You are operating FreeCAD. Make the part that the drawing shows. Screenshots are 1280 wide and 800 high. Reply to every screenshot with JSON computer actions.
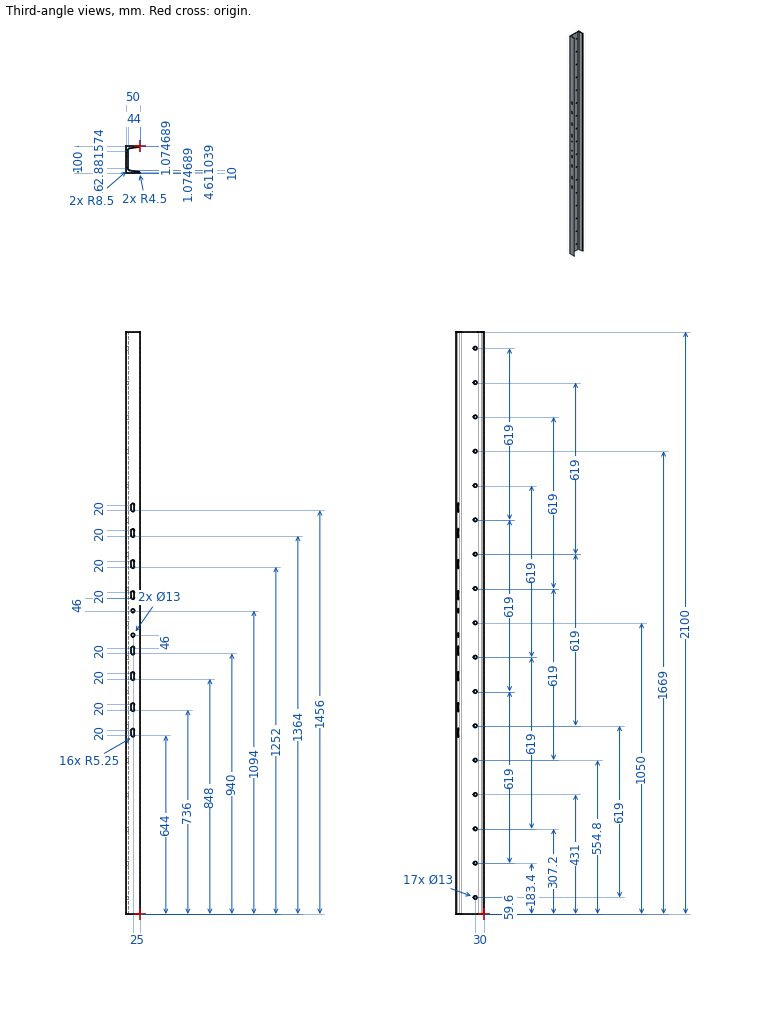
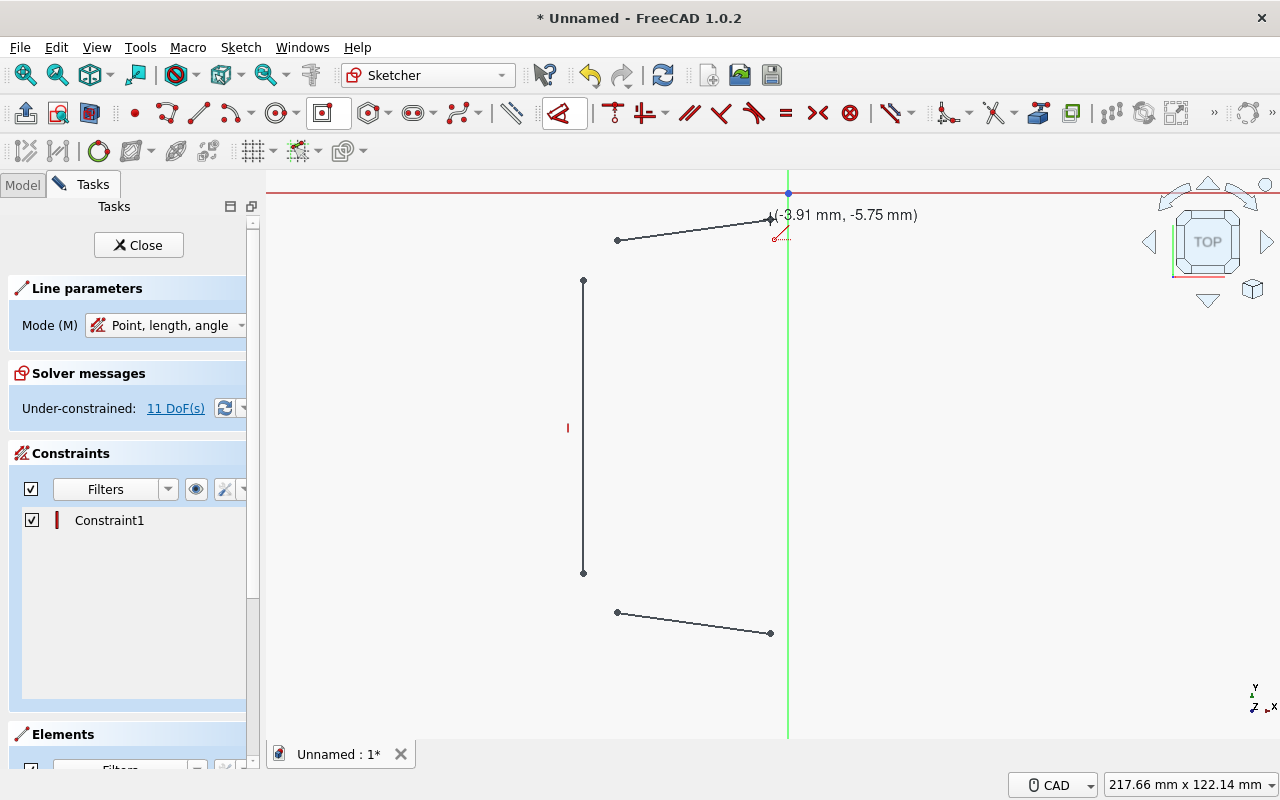
{"action": "left_click", "coordinate": [168, 114]}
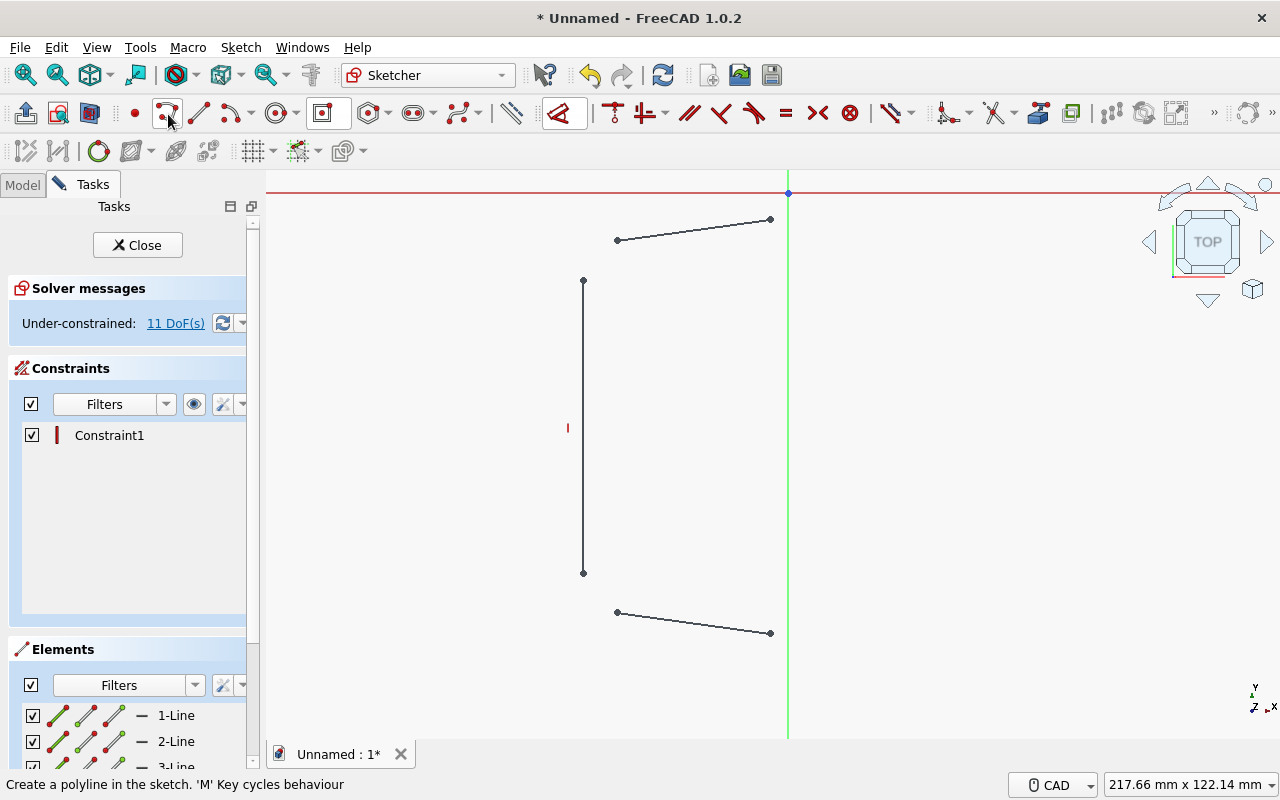
{"action": "scroll", "coordinate": [788, 198], "scroll_direction": "up", "scroll_amount": 6}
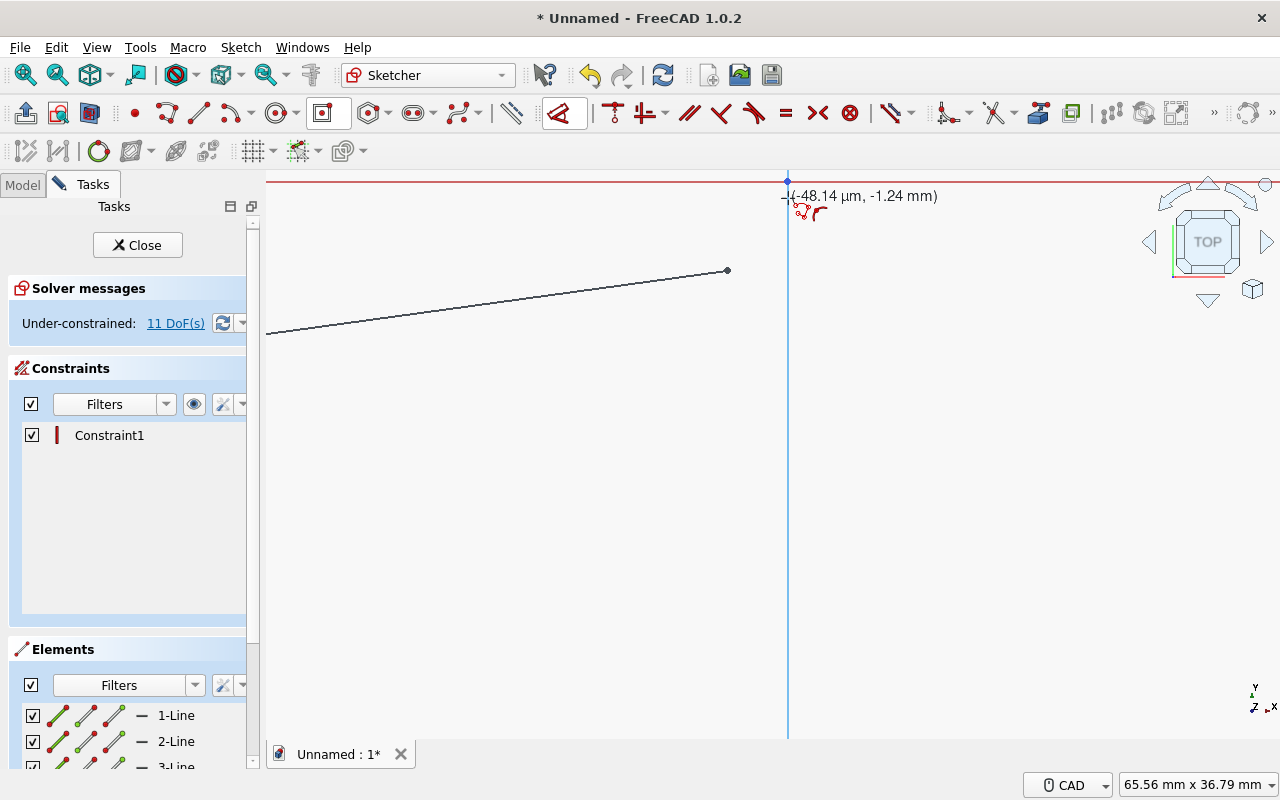
{"action": "left_click", "coordinate": [788, 199]}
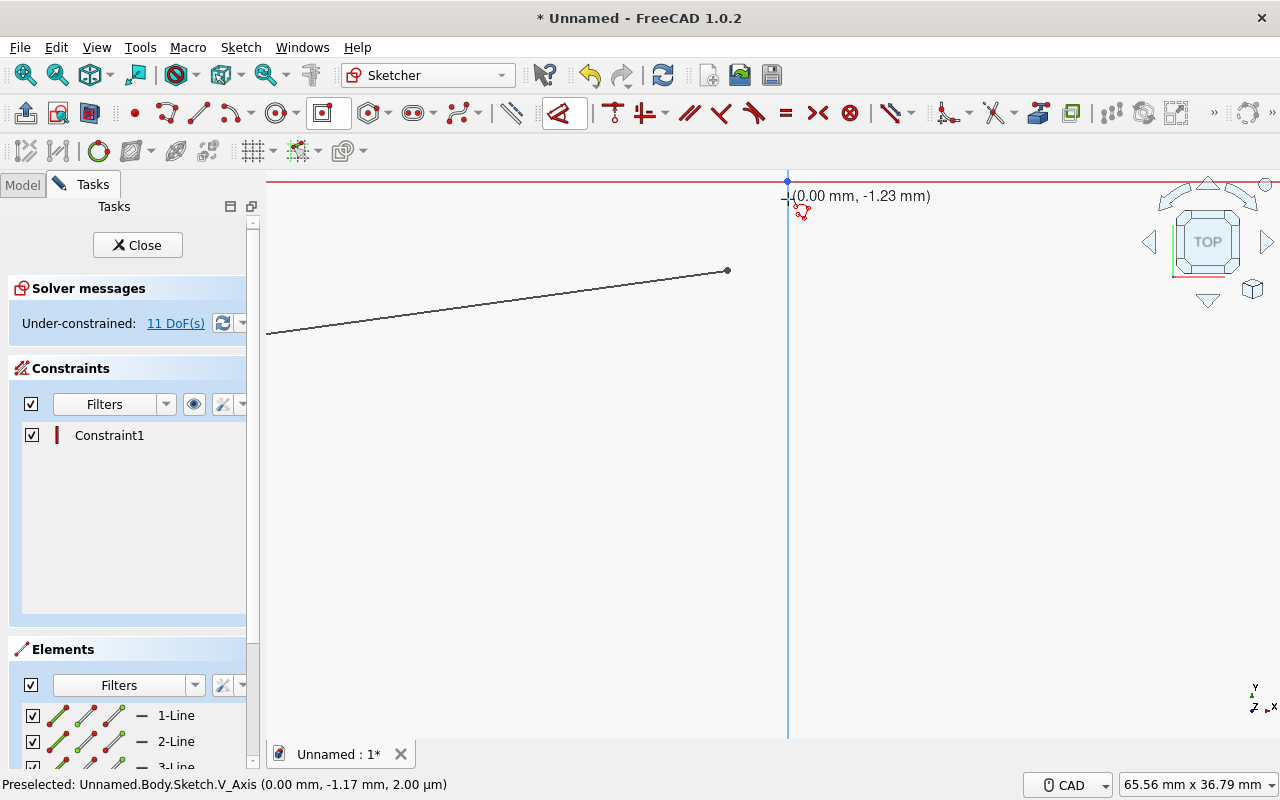
{"action": "scroll", "coordinate": [804, 291], "scroll_direction": "down", "scroll_amount": 7}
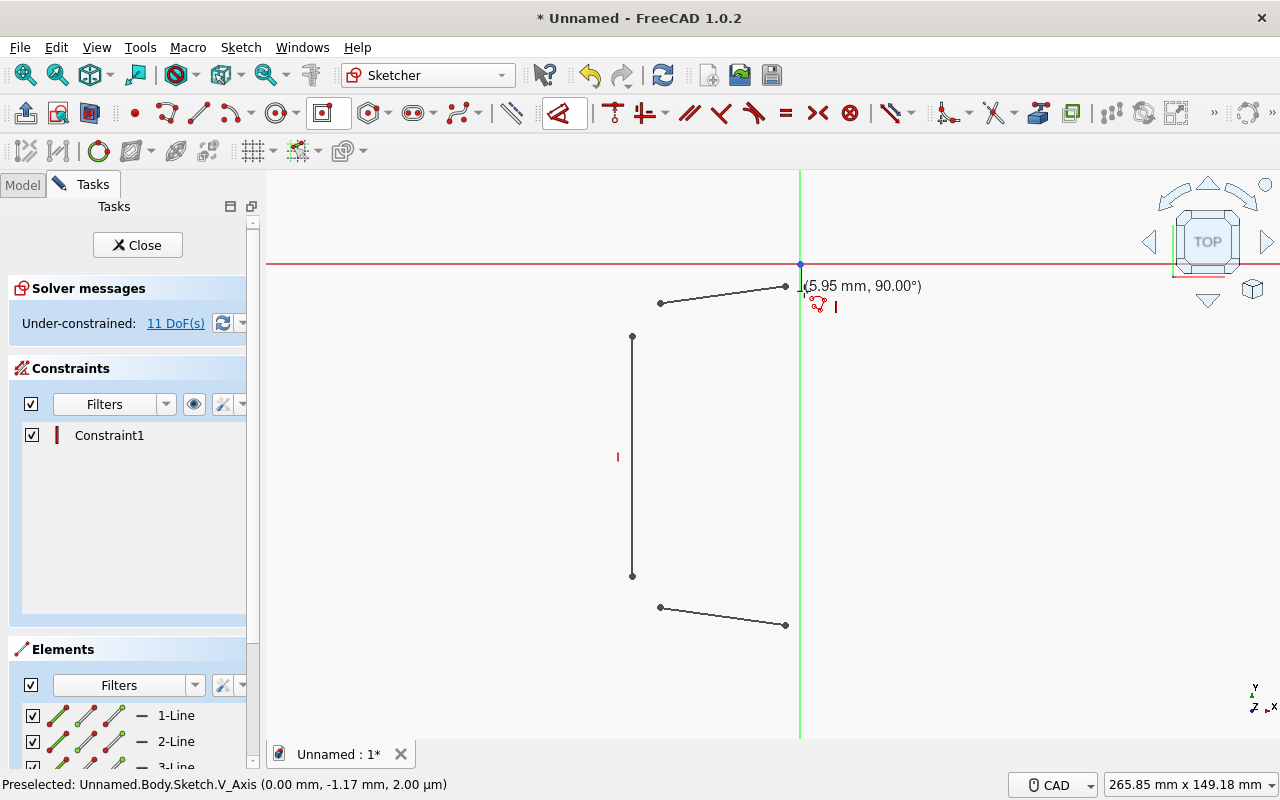
{"action": "scroll", "coordinate": [800, 264], "scroll_direction": "up", "scroll_amount": 7}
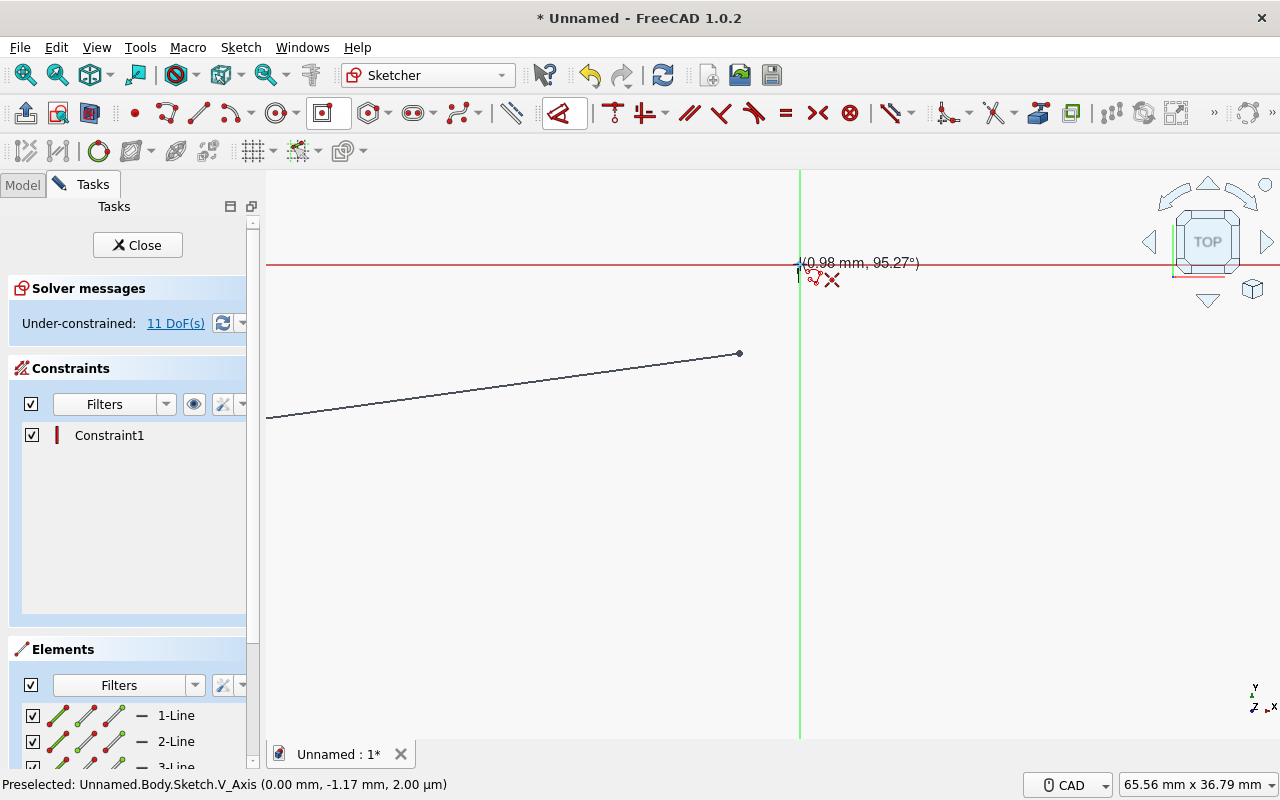
{"action": "left_click", "coordinate": [800, 265]}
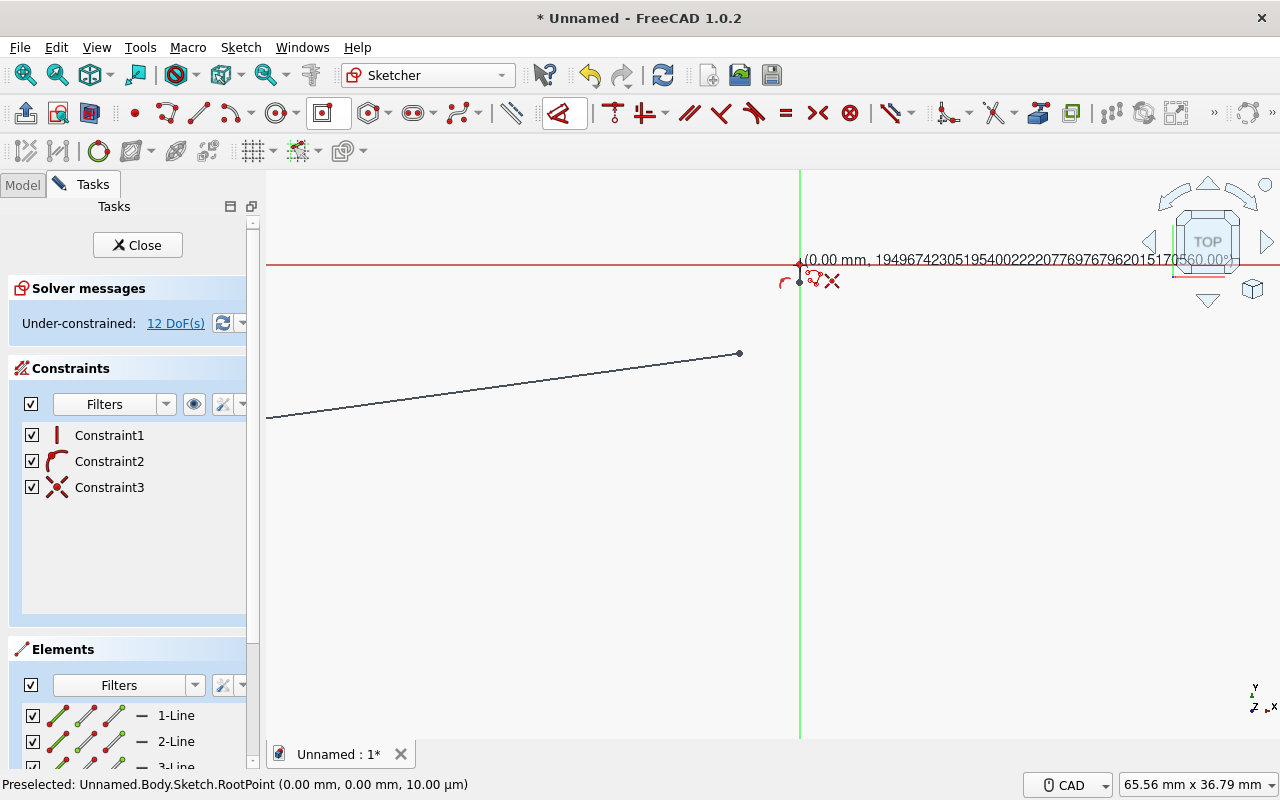
{"action": "scroll", "coordinate": [800, 264], "scroll_direction": "down", "scroll_amount": 7}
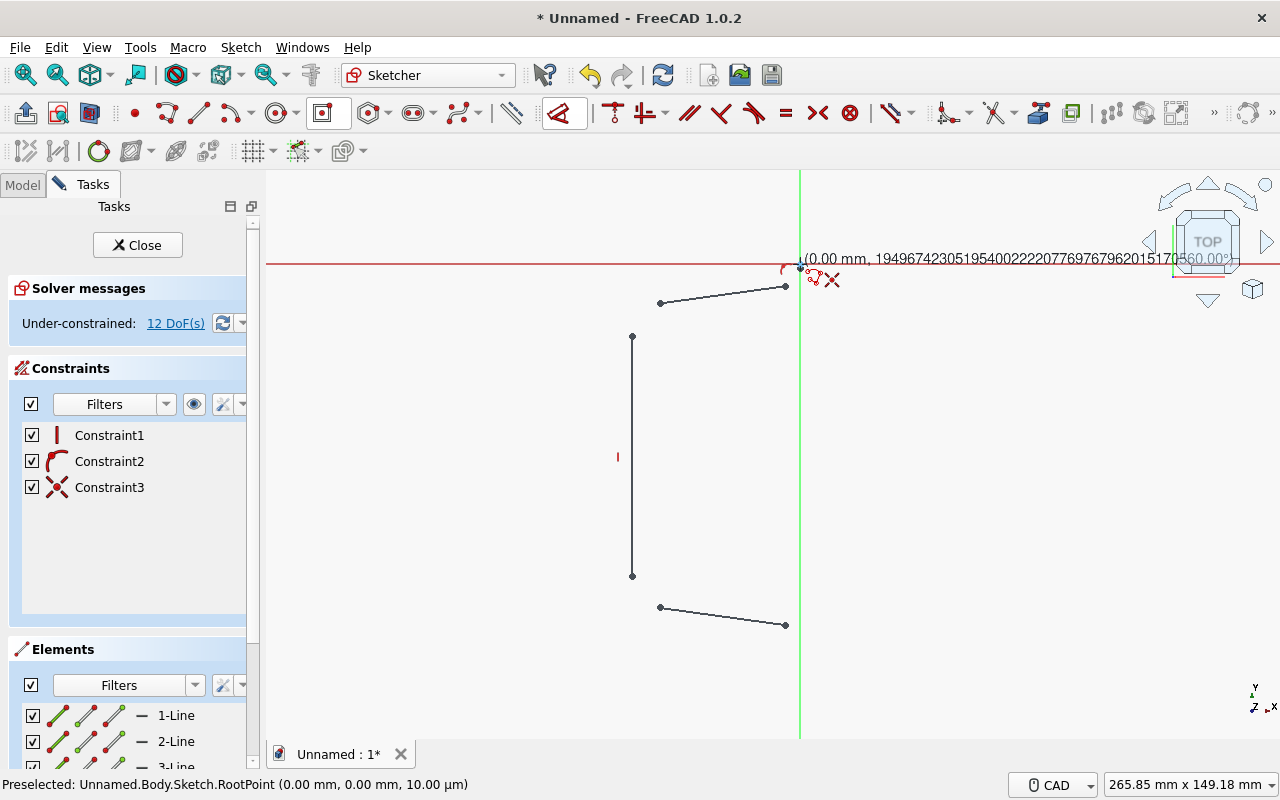
{"action": "left_click", "coordinate": [610, 273]}
{"action": "left_click", "coordinate": [610, 646]}
{"action": "left_click", "coordinate": [800, 646]}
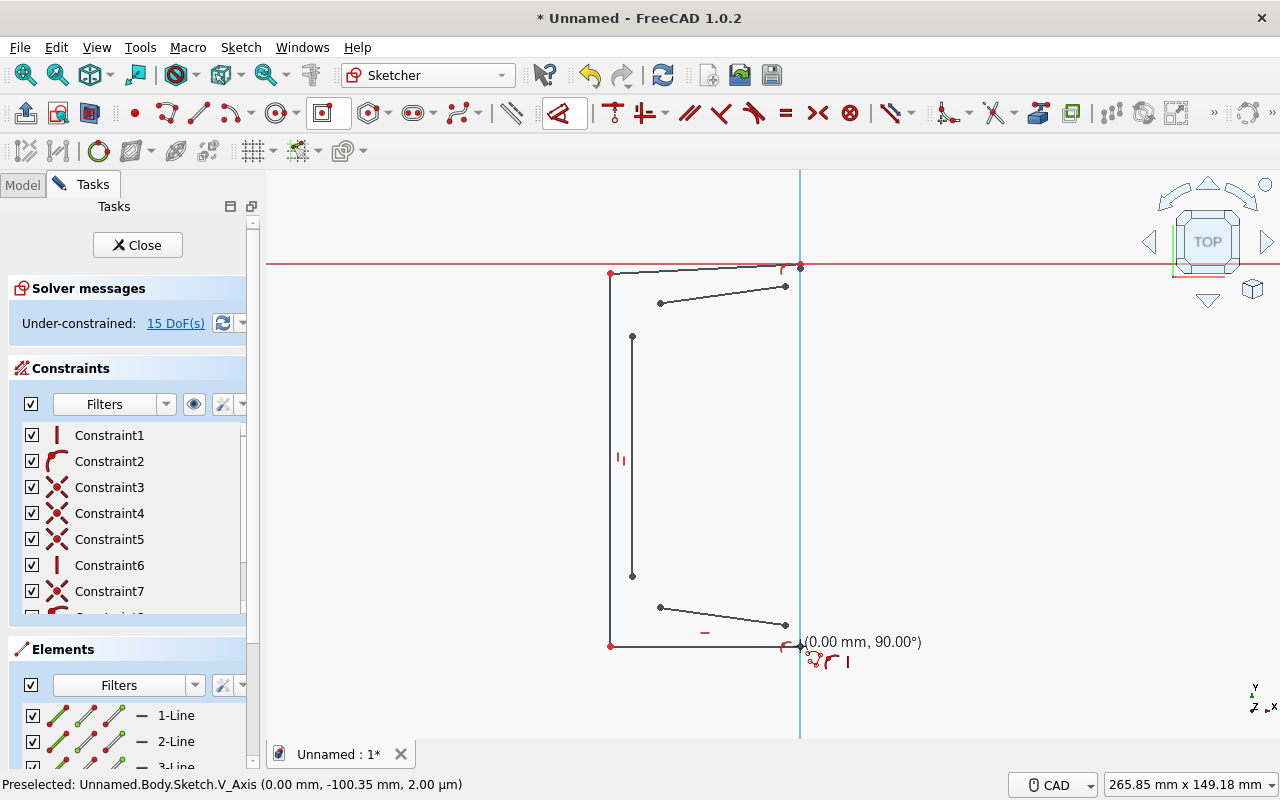
{"action": "scroll", "coordinate": [800, 642], "scroll_direction": "up", "scroll_amount": 7}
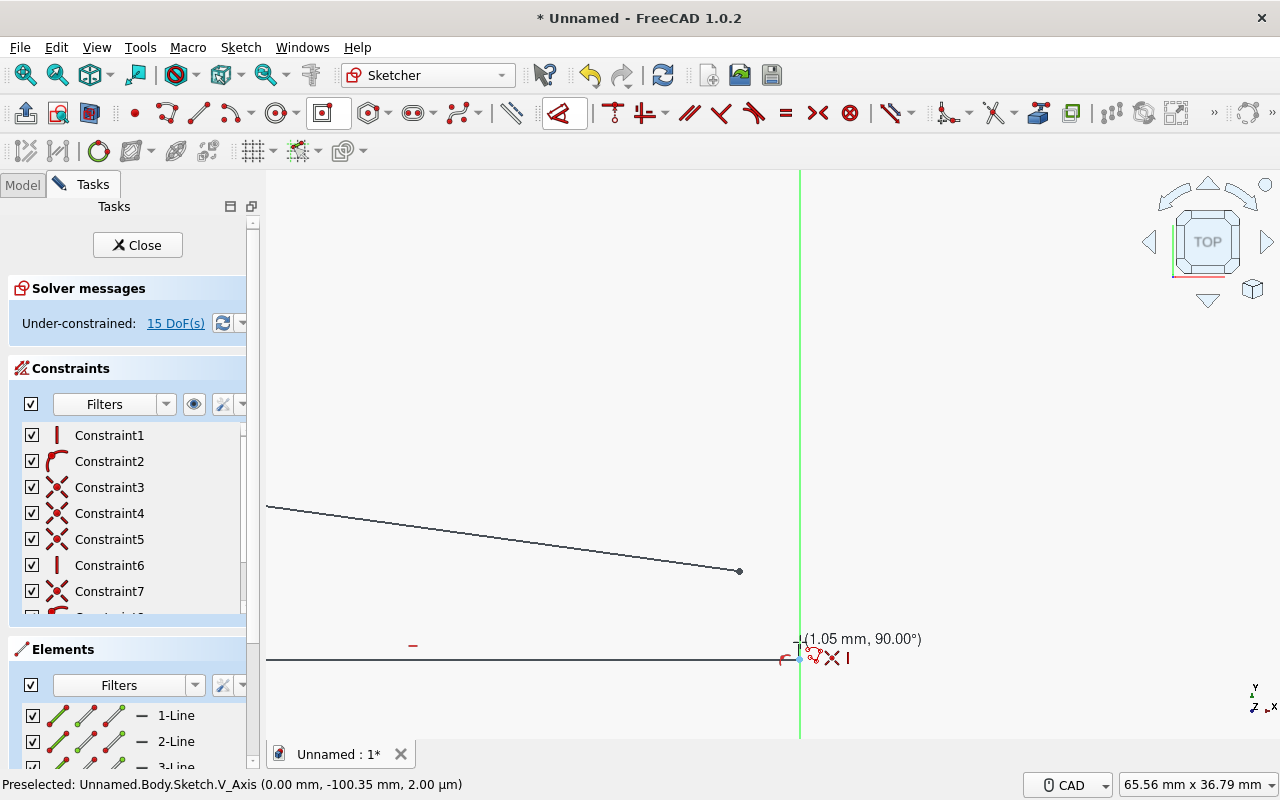
{"action": "left_click", "coordinate": [791, 638]}
{"action": "right_click", "coordinate": [791, 638]}